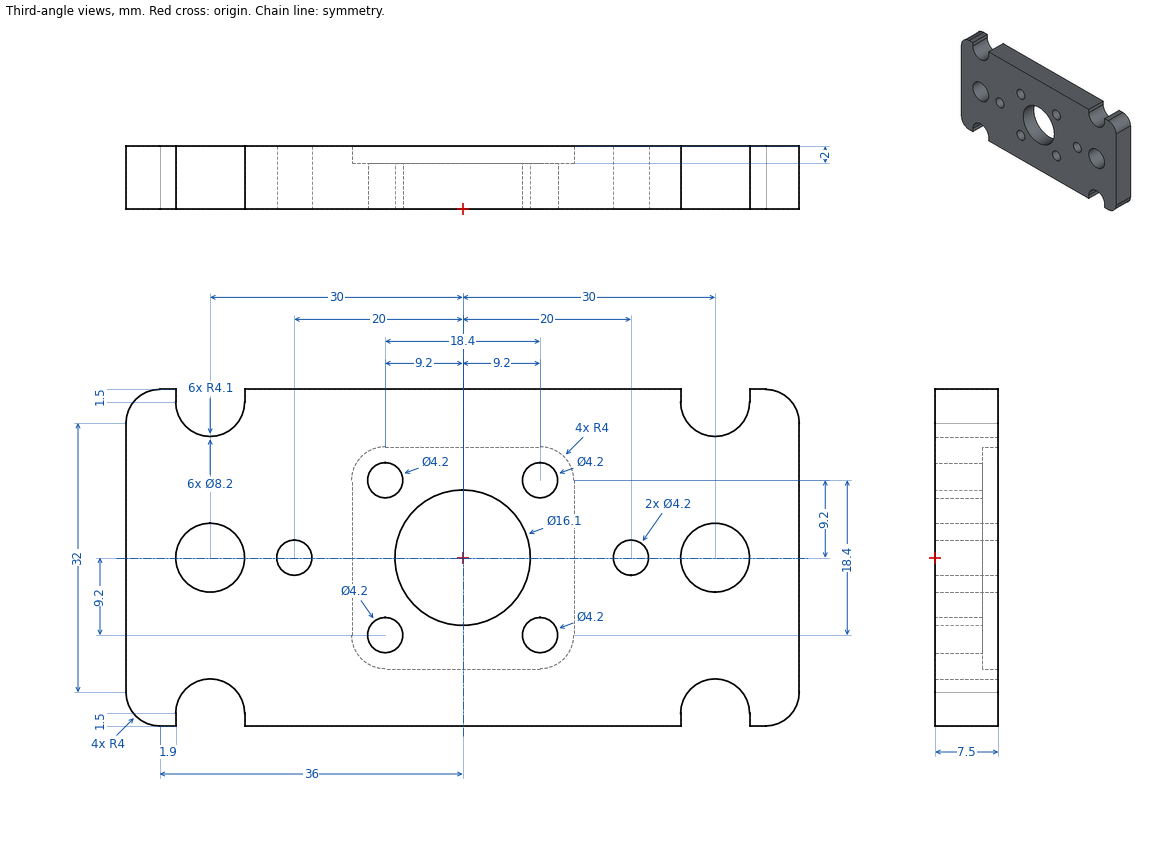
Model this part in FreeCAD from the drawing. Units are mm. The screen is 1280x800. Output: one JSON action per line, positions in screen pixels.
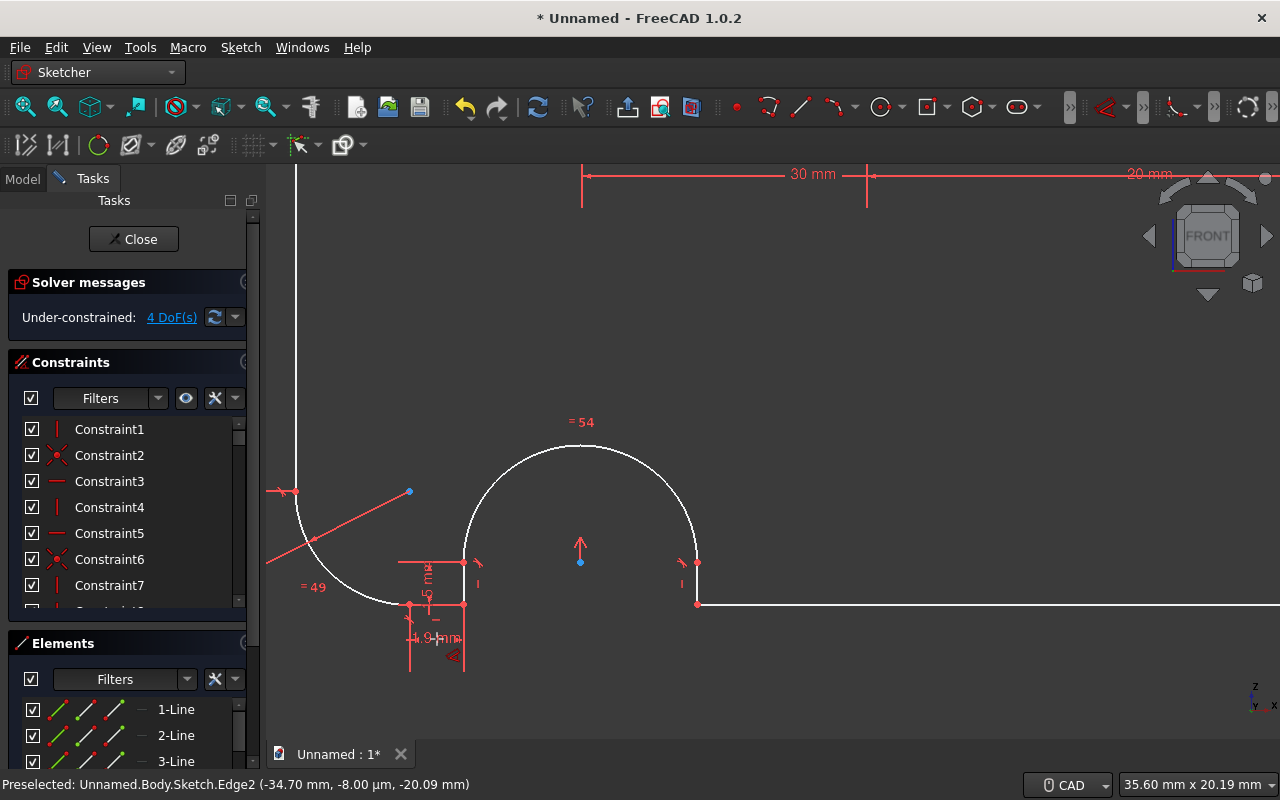
{"action": "scroll", "coordinate": [465, 589], "scroll_direction": "down", "scroll_amount": 7}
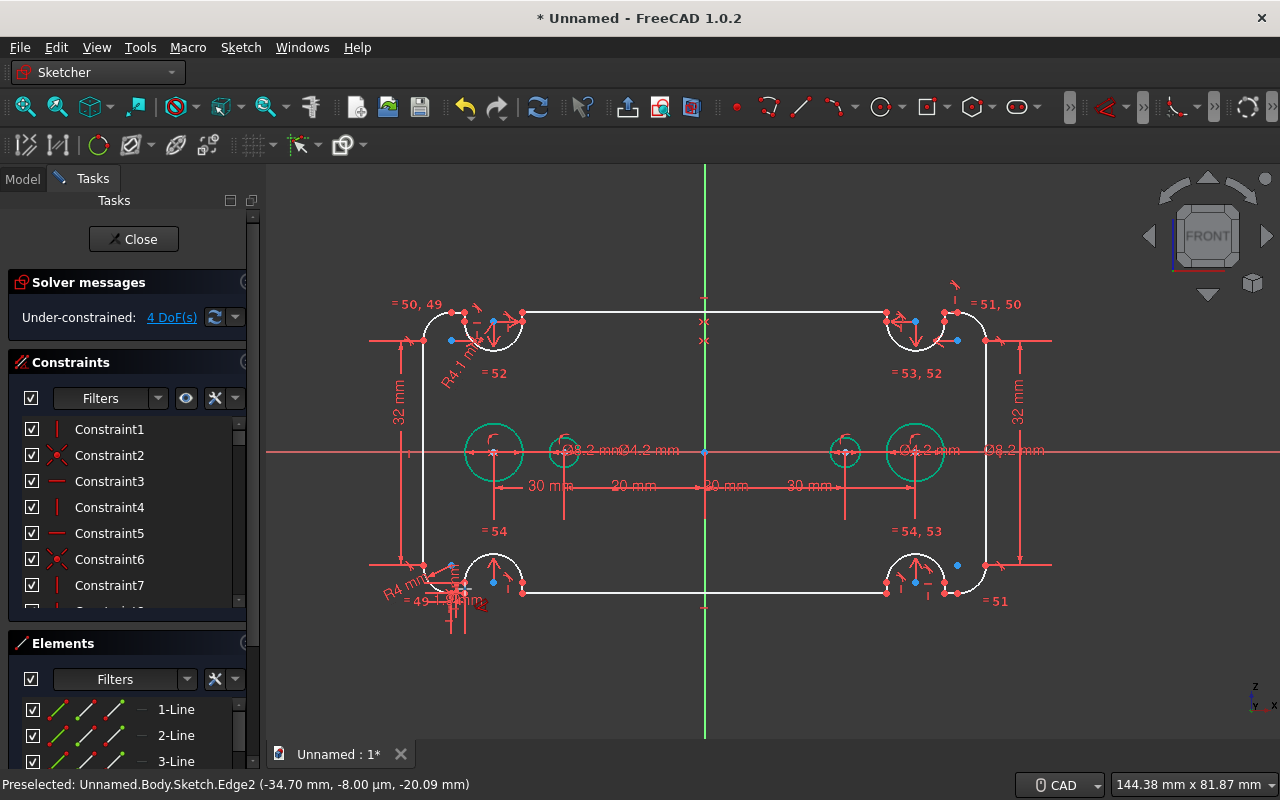
{"action": "scroll", "coordinate": [465, 315], "scroll_direction": "up", "scroll_amount": 8}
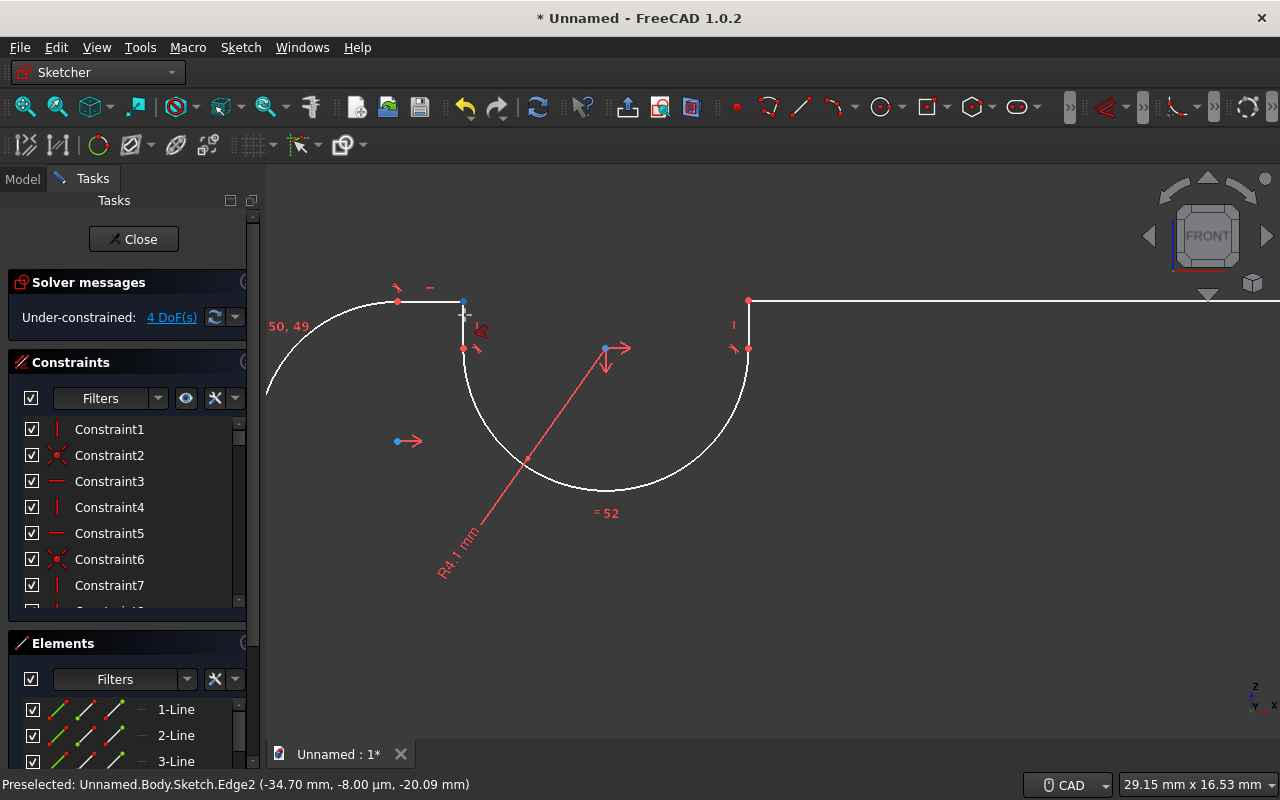
{"action": "left_click", "coordinate": [463, 316]}
{"action": "left_click", "coordinate": [429, 325]}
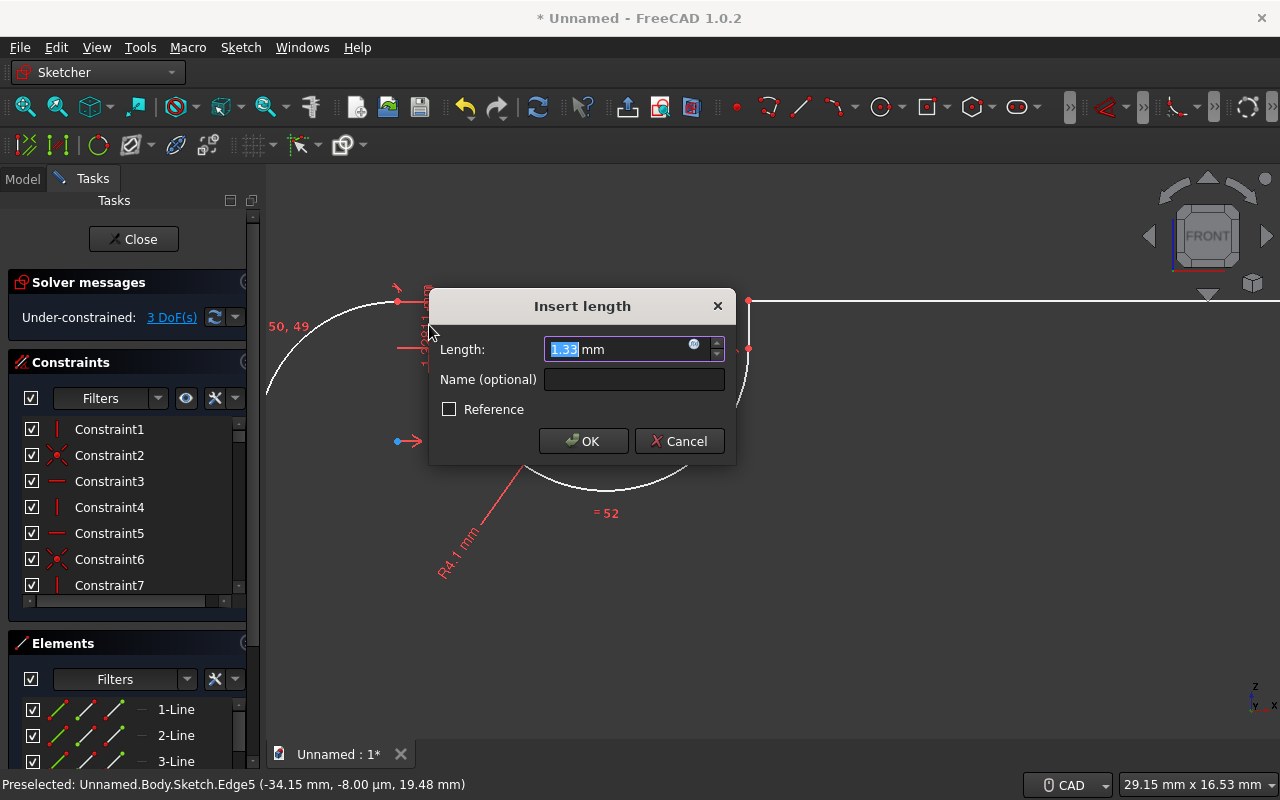
{"action": "type", "text": "1.5"}
{"action": "key", "text": "Return"}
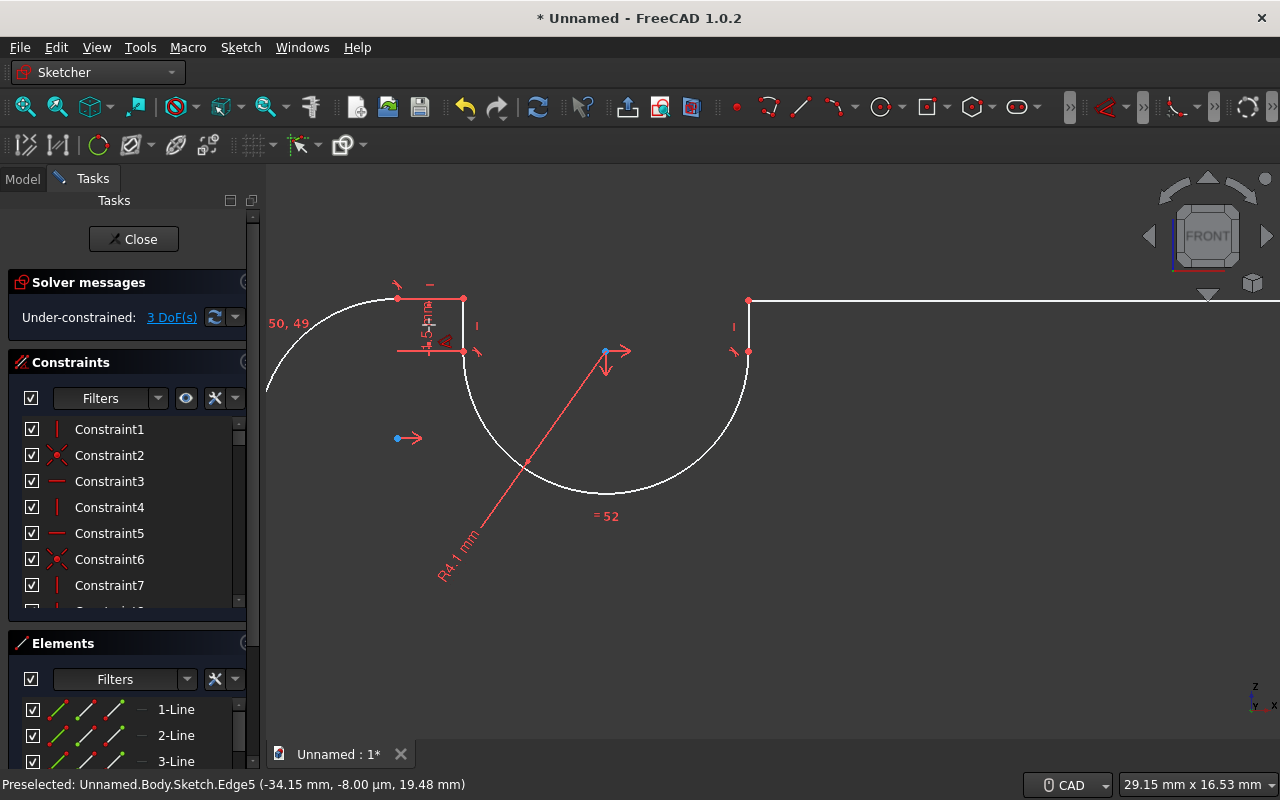
{"action": "left_click", "coordinate": [749, 336]}
{"action": "left_click", "coordinate": [715, 326]}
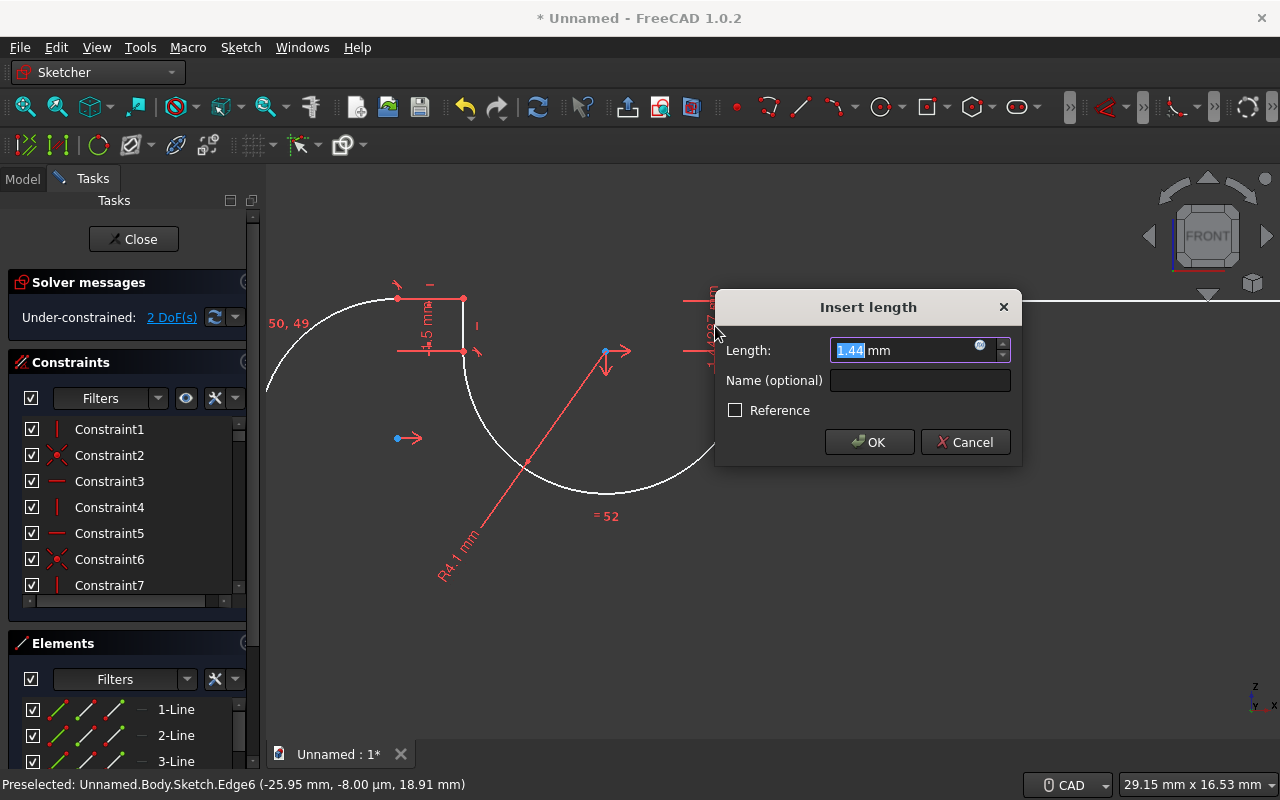
{"action": "type", "text": "1.5"}
{"action": "key", "text": "Return"}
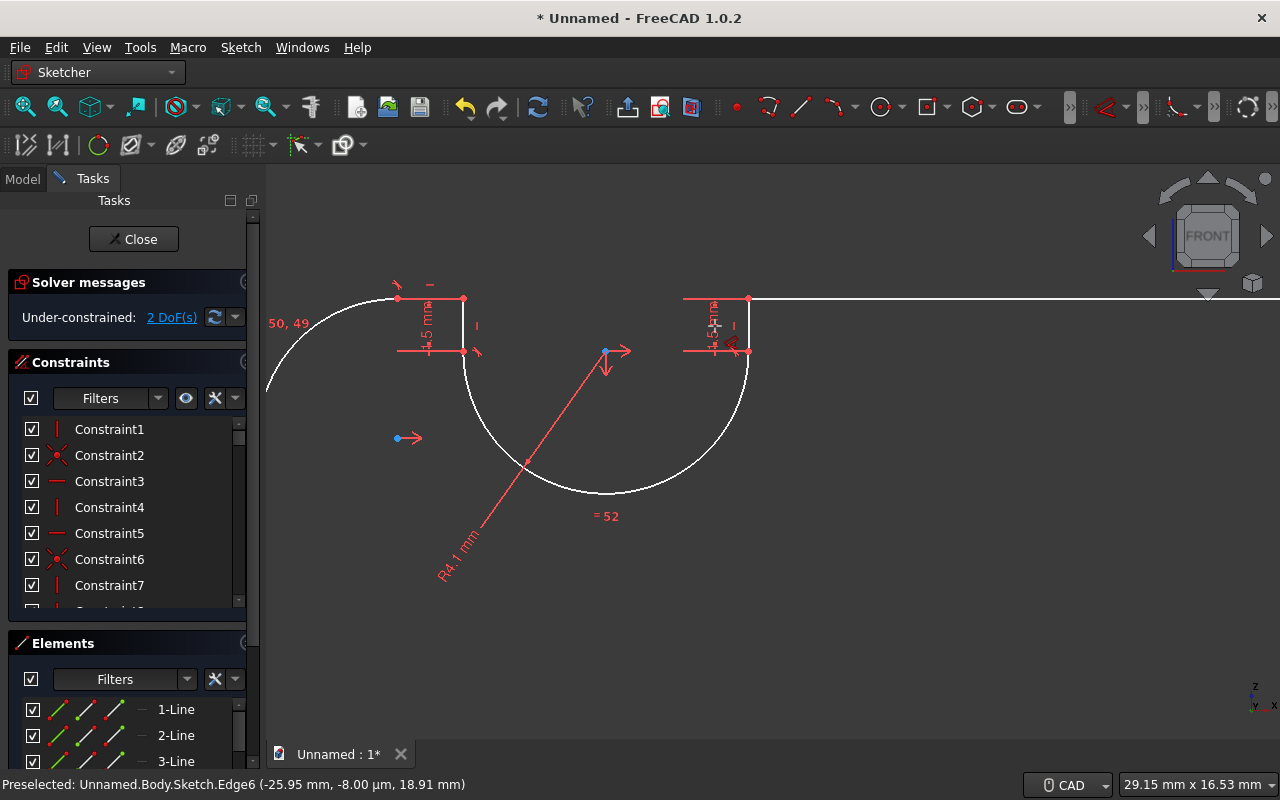
{"action": "scroll", "coordinate": [465, 314], "scroll_direction": "down", "scroll_amount": 8}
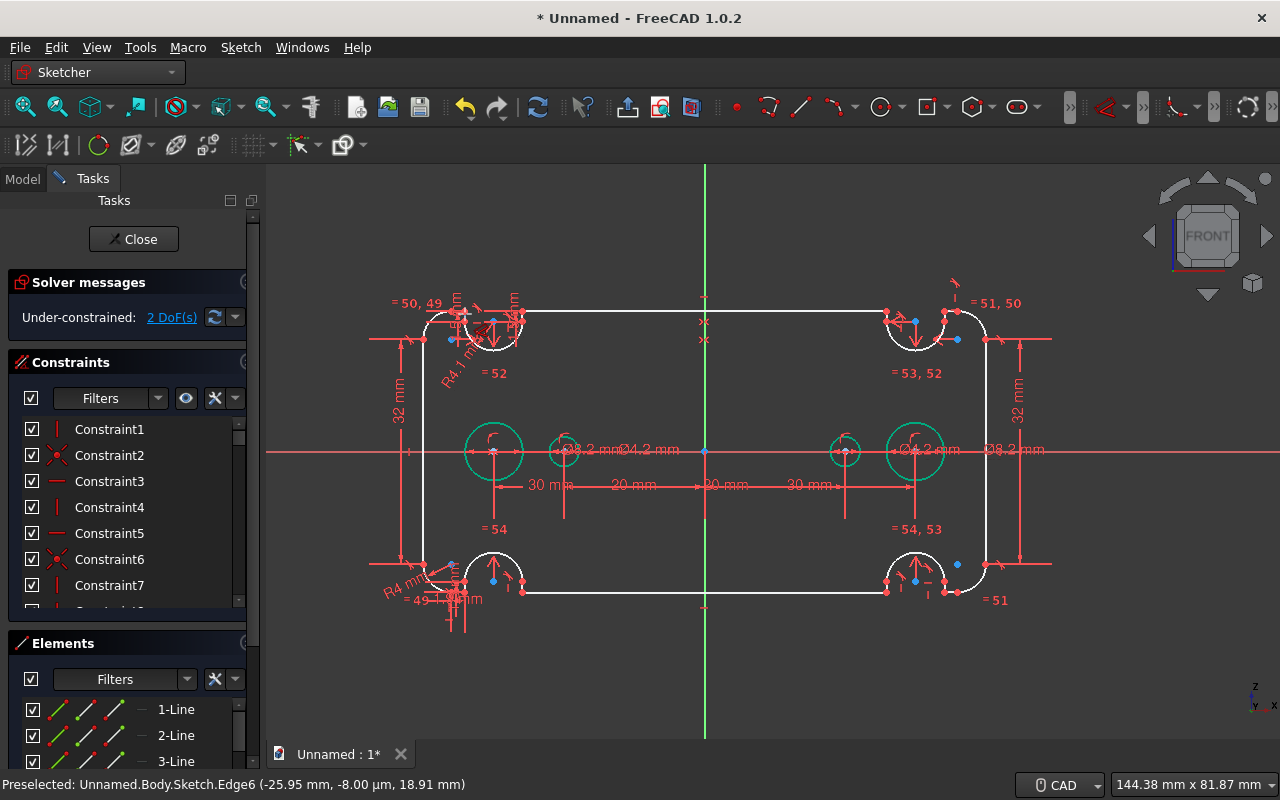
{"action": "scroll", "coordinate": [887, 585], "scroll_direction": "up", "scroll_amount": 8}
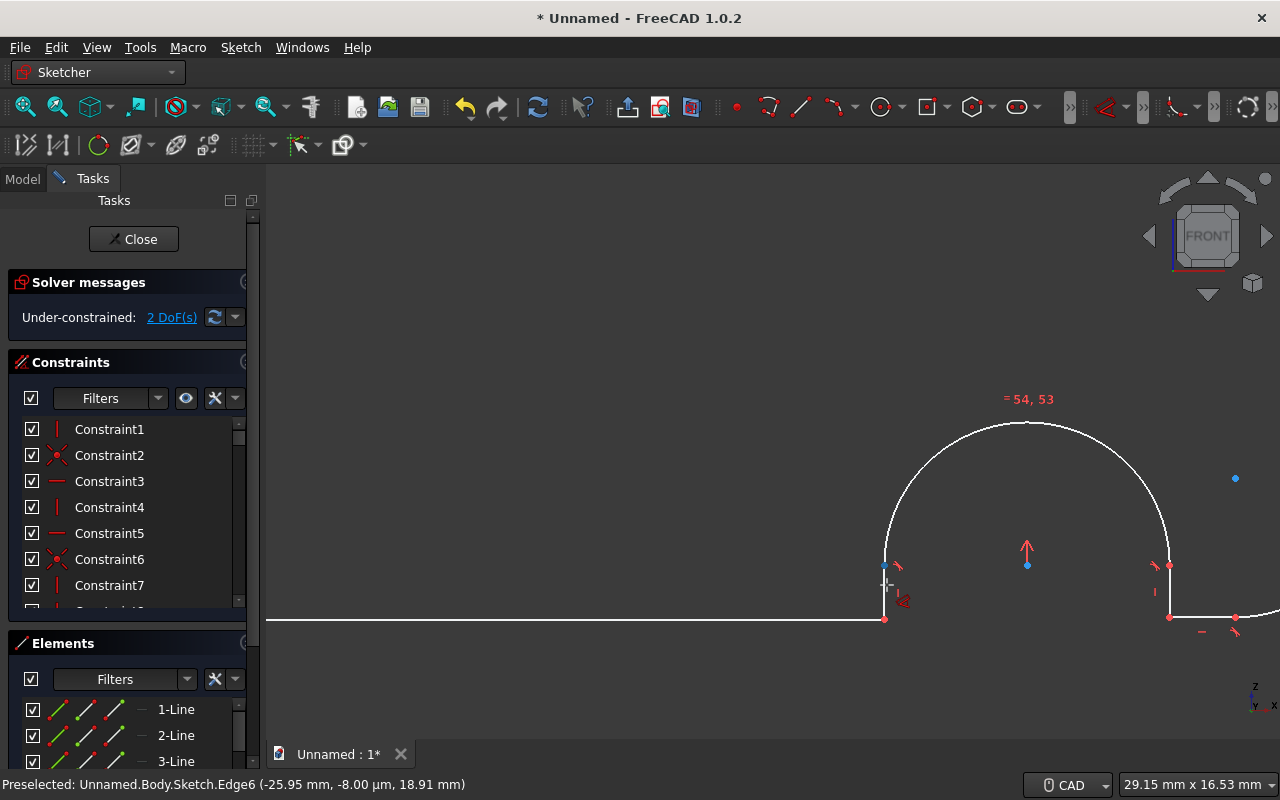
{"action": "left_click", "coordinate": [884, 582]}
{"action": "left_click", "coordinate": [918, 592]}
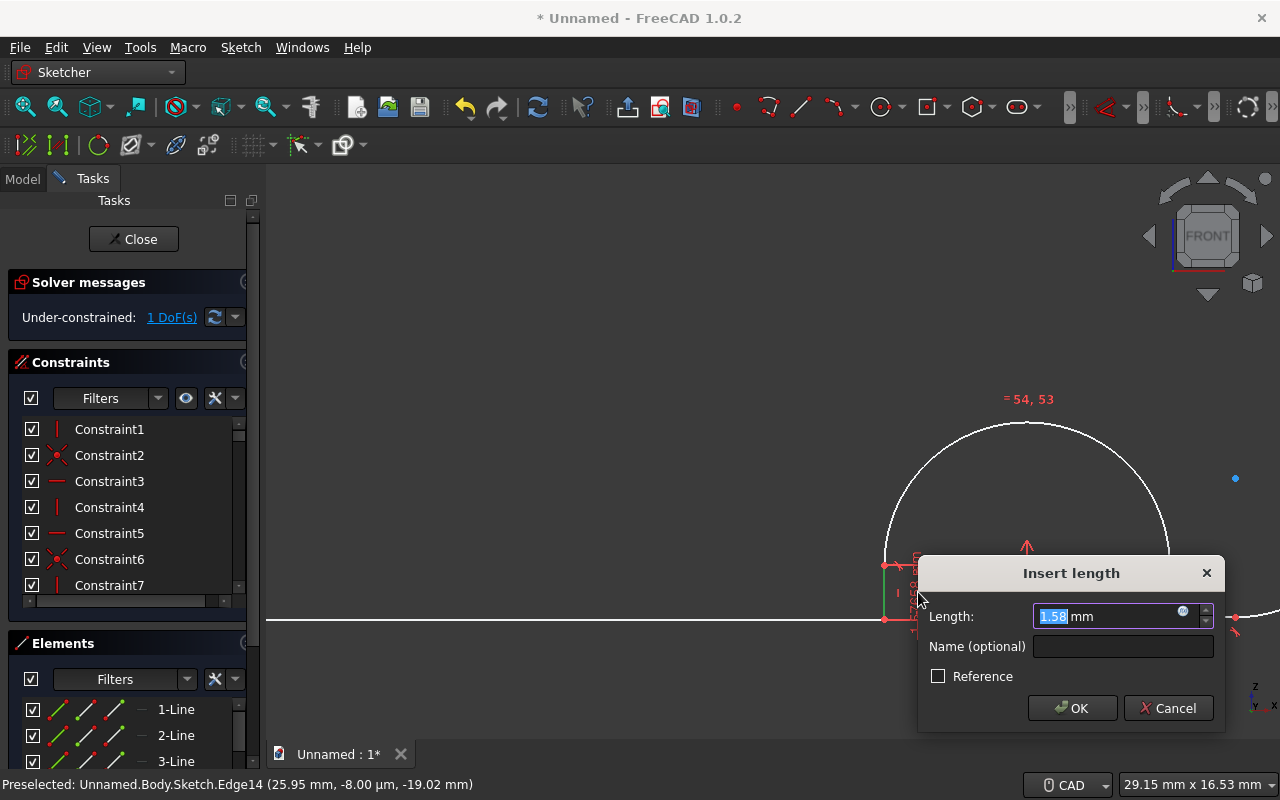
{"action": "type", "text": "1.5"}
{"action": "key", "text": "Return"}